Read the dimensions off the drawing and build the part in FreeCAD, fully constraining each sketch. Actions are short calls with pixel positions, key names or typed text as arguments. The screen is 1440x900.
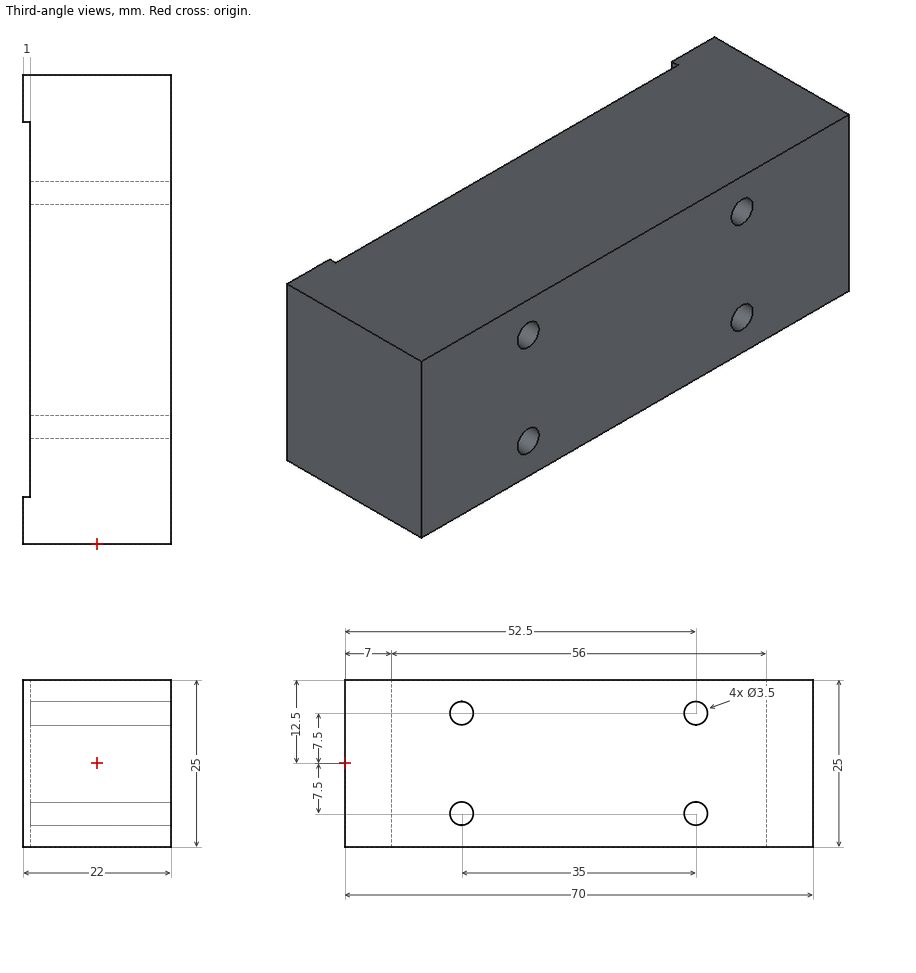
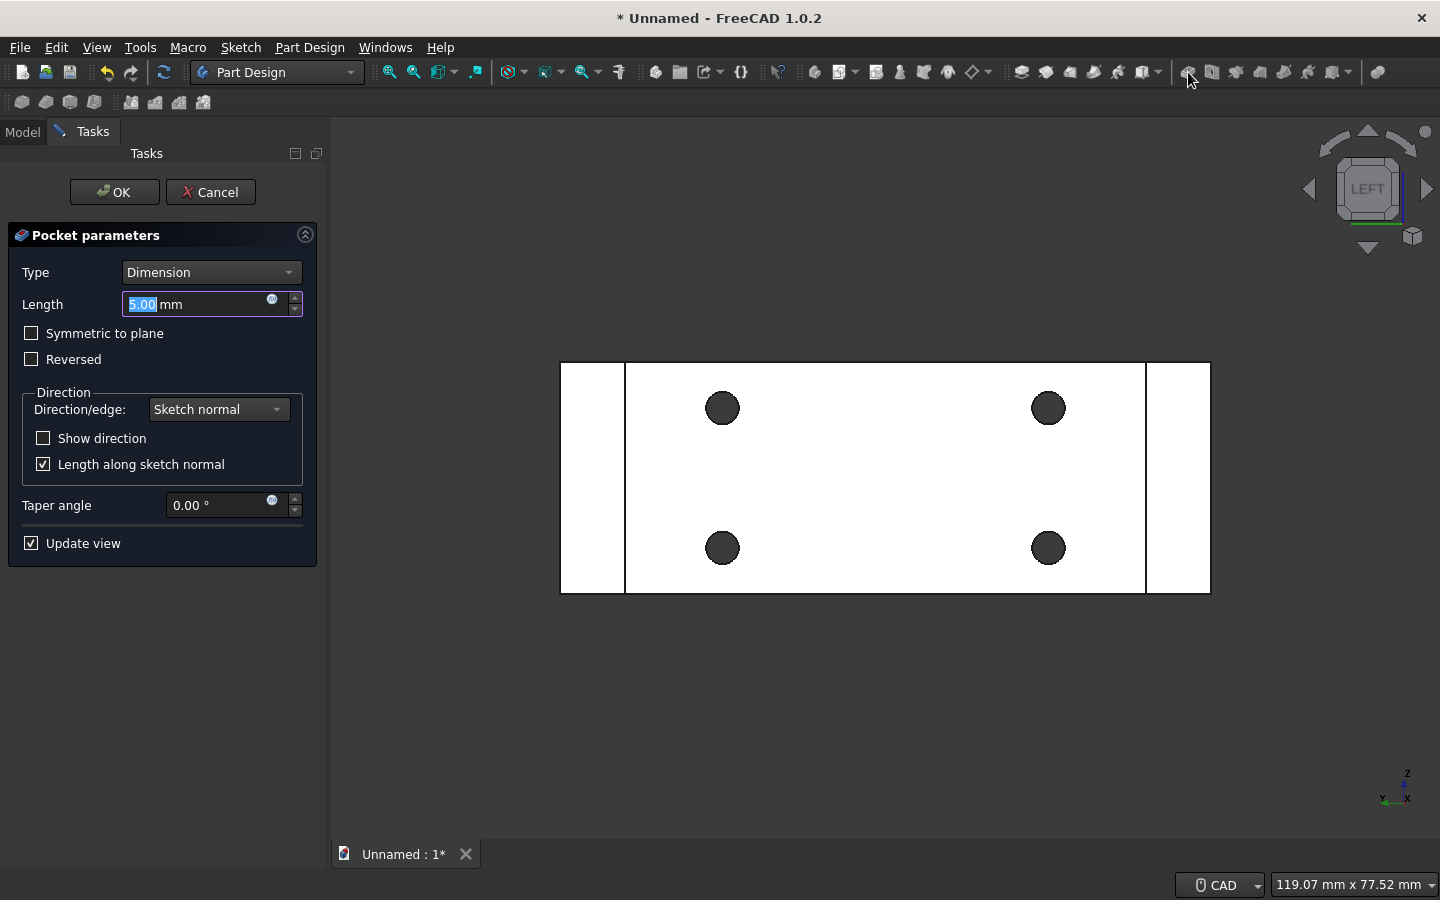
text(1)
key(Tab)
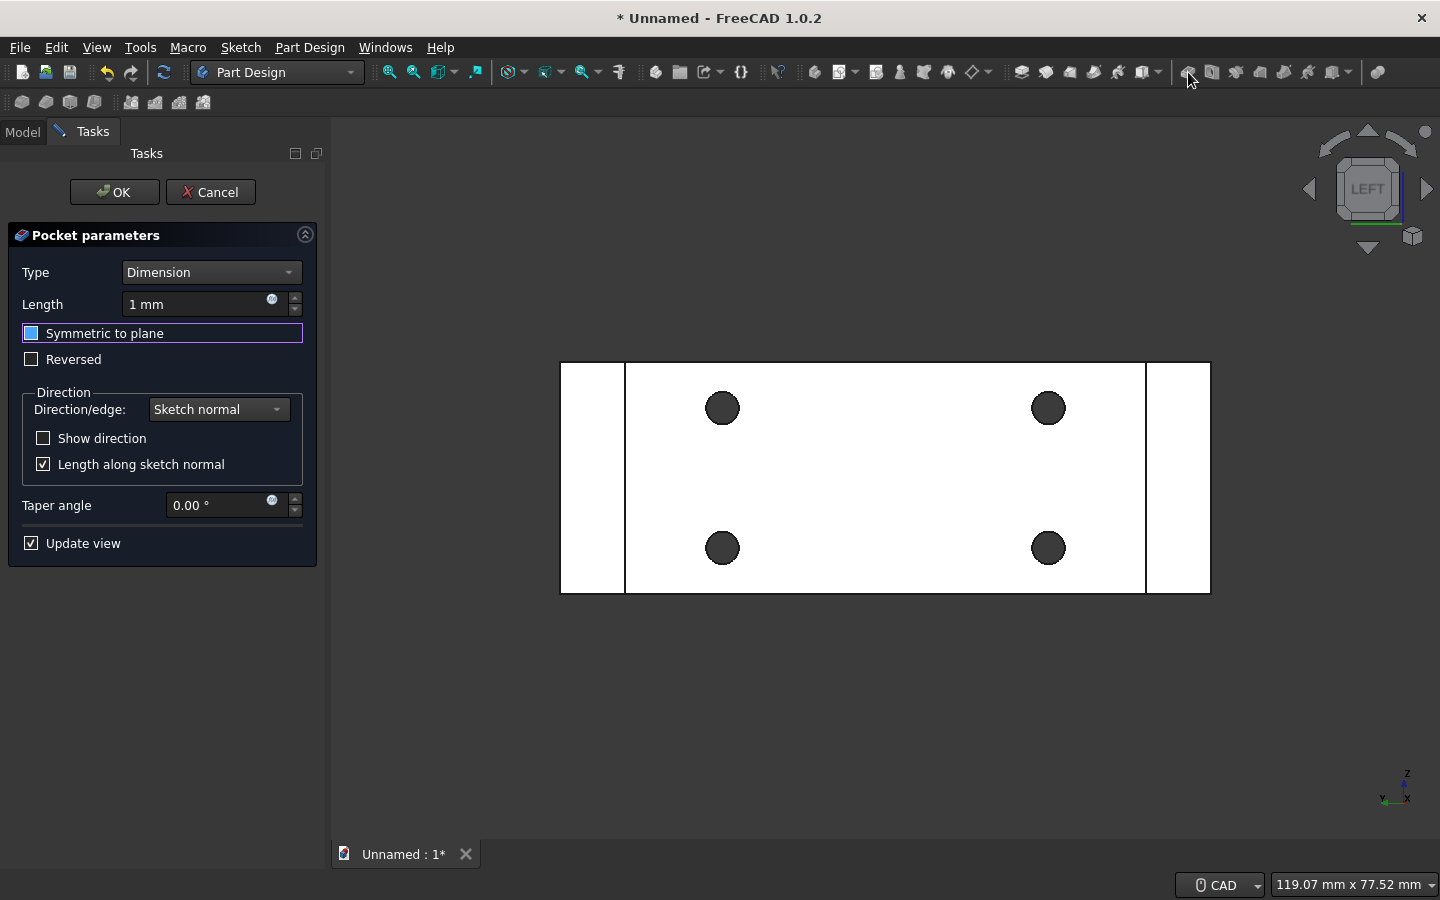
click(115, 192)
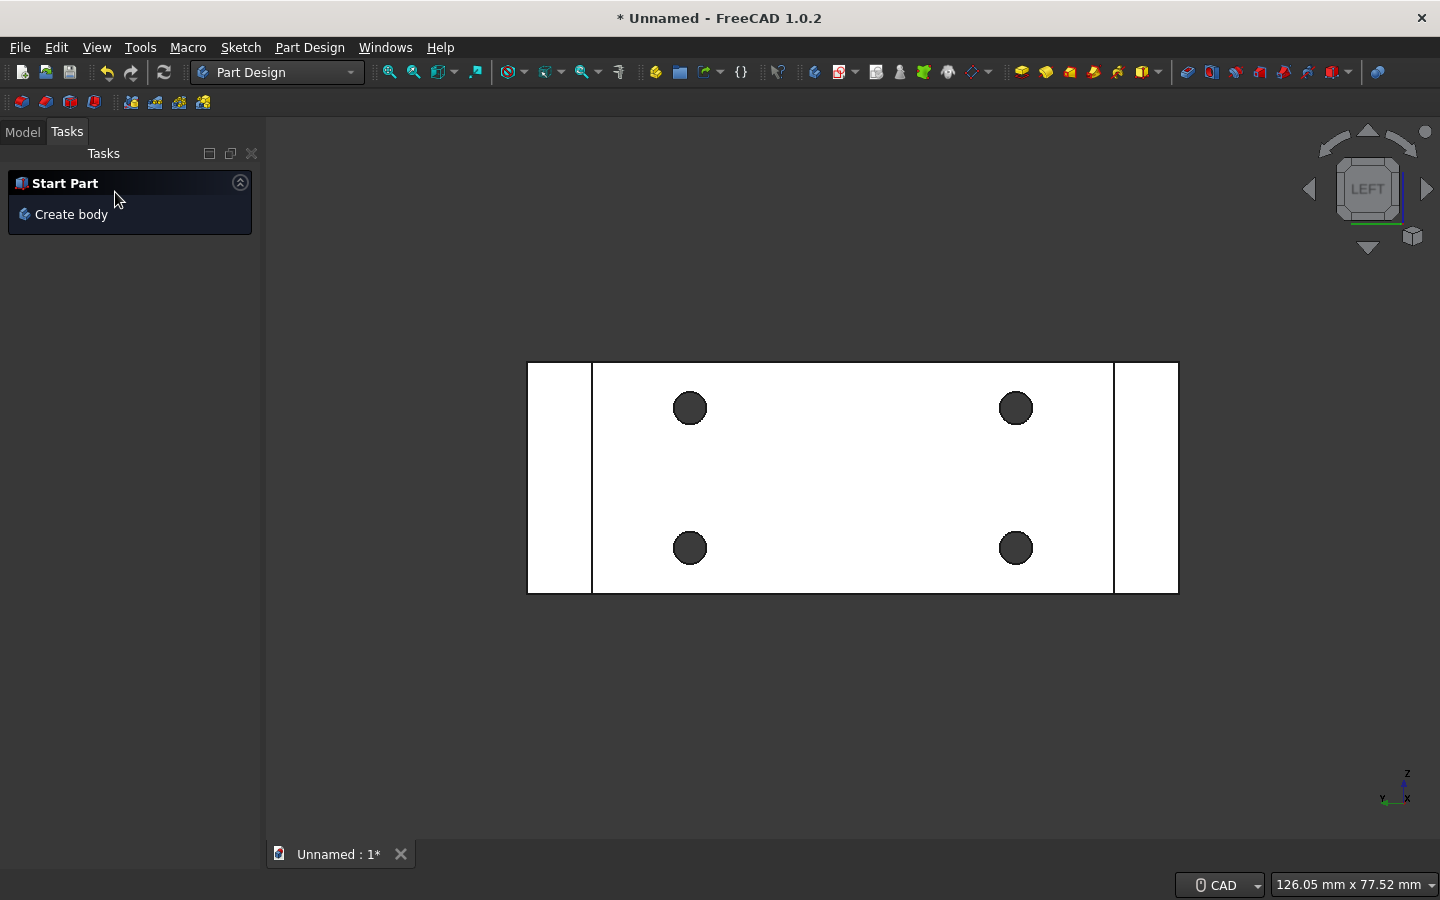
key(0)